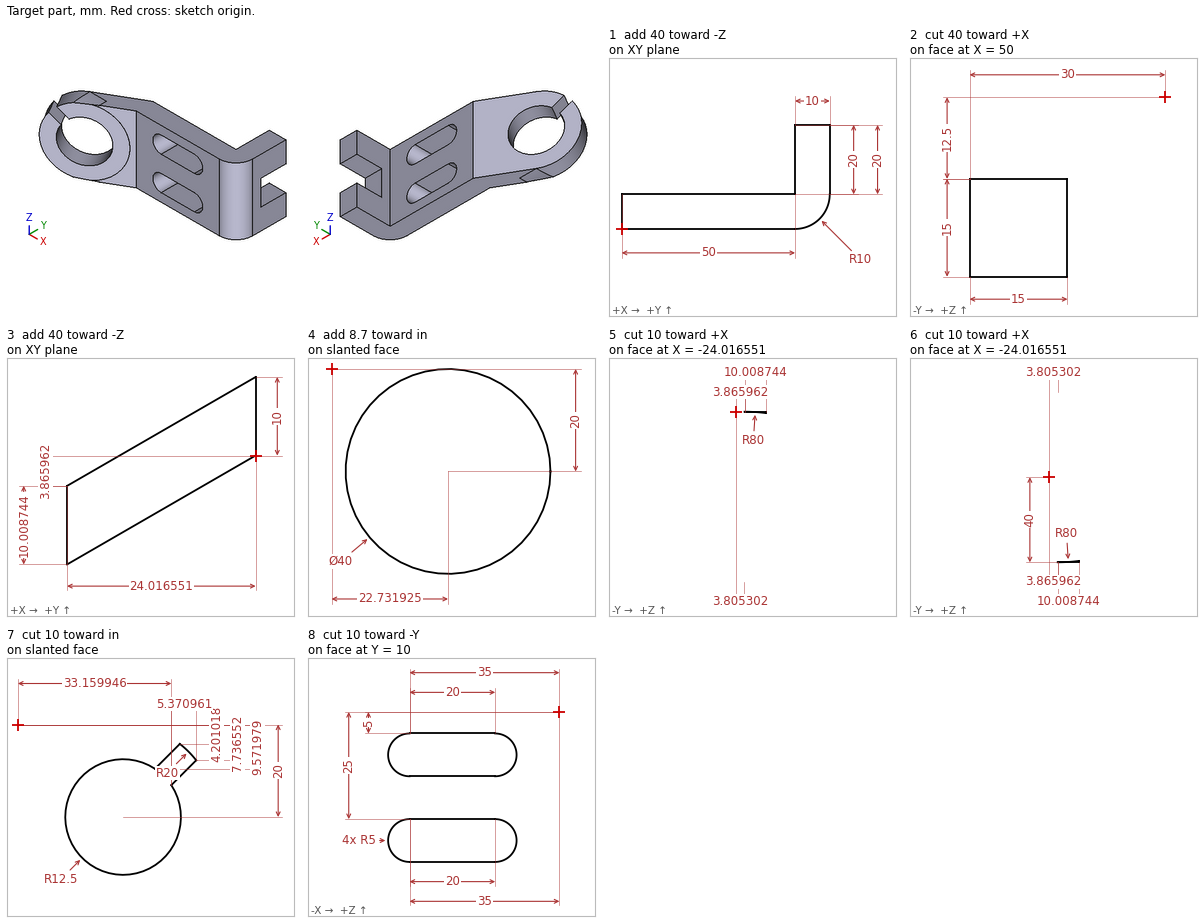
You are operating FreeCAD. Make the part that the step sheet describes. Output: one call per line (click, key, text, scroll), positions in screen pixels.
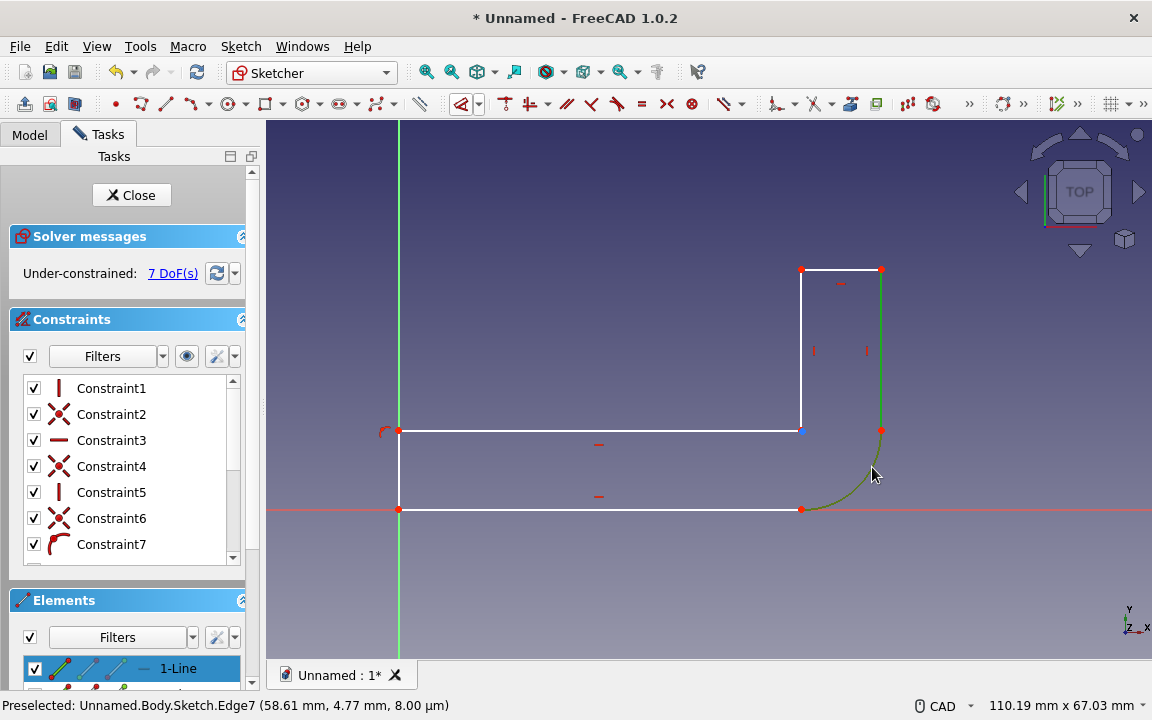
click(617, 104)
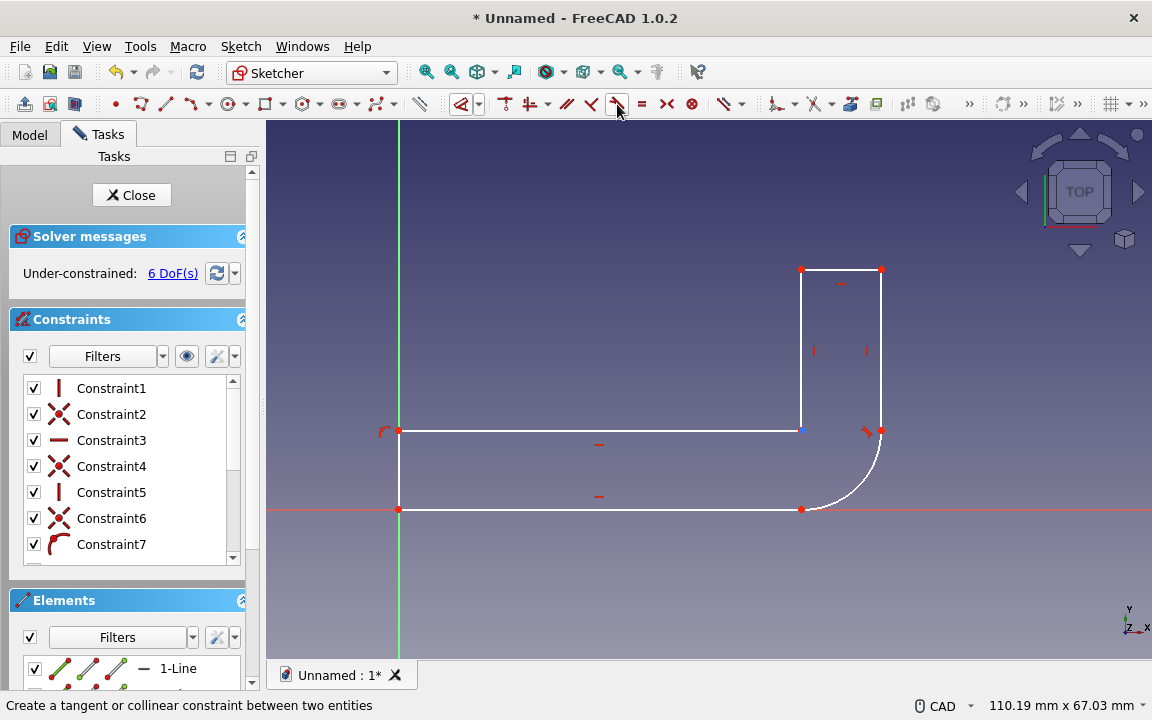
click(519, 510)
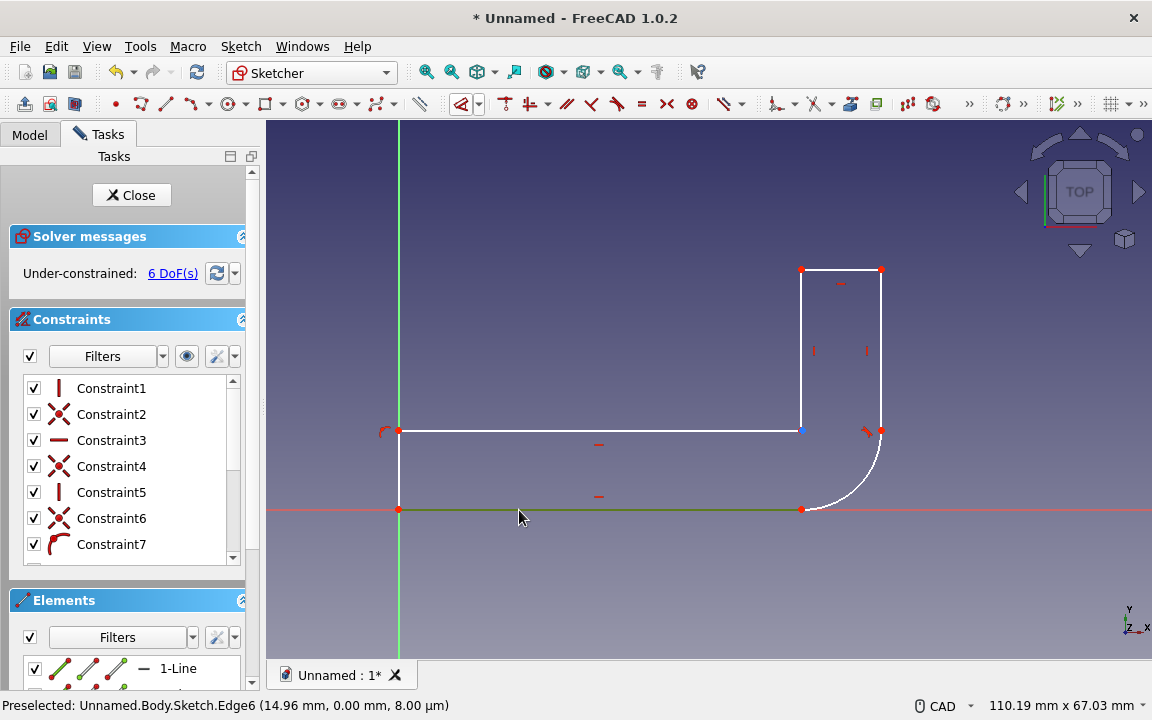
click(872, 467)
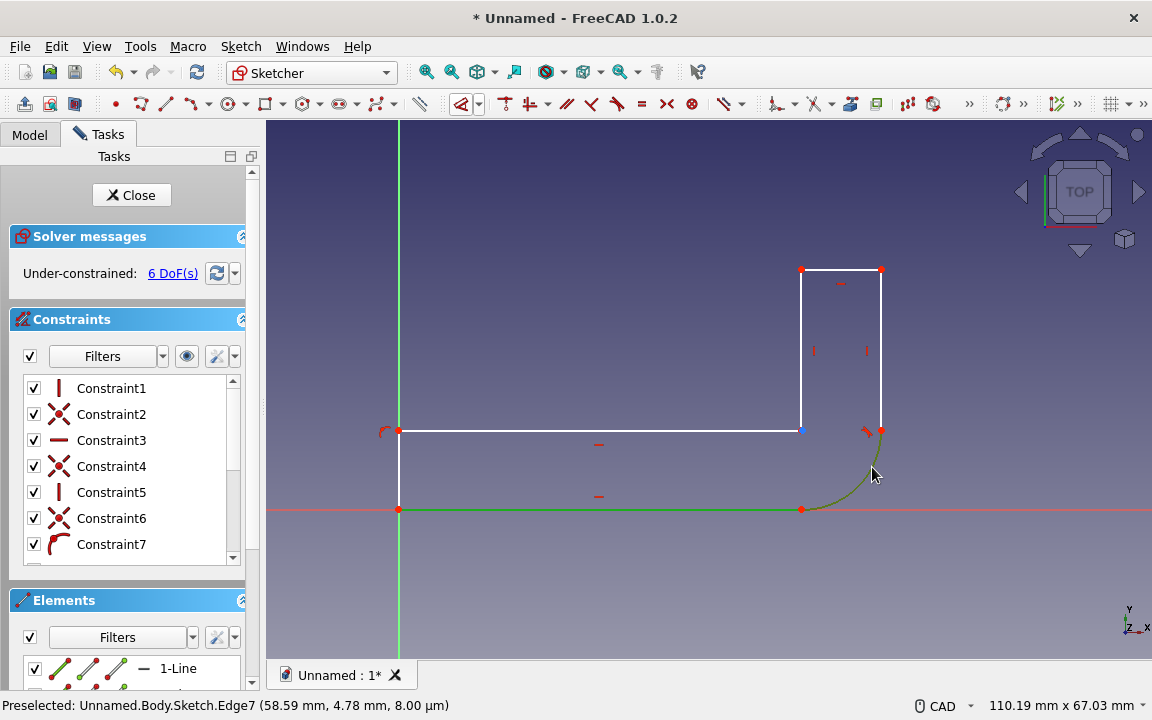
click(617, 104)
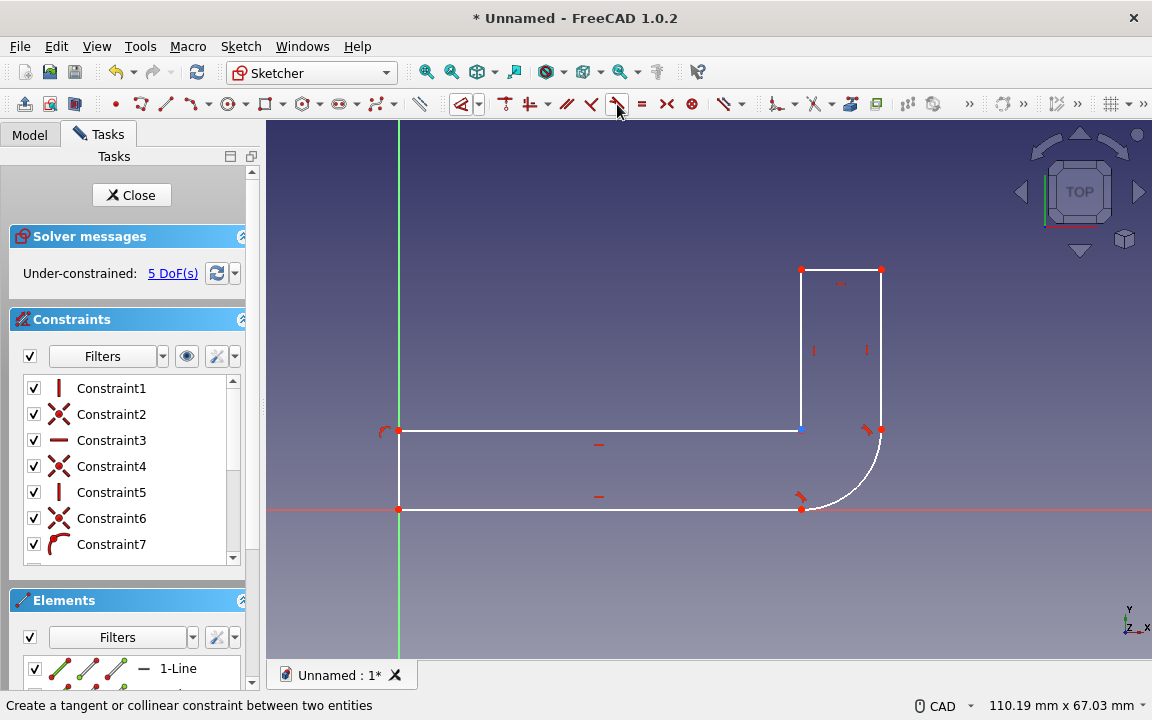
click(872, 466)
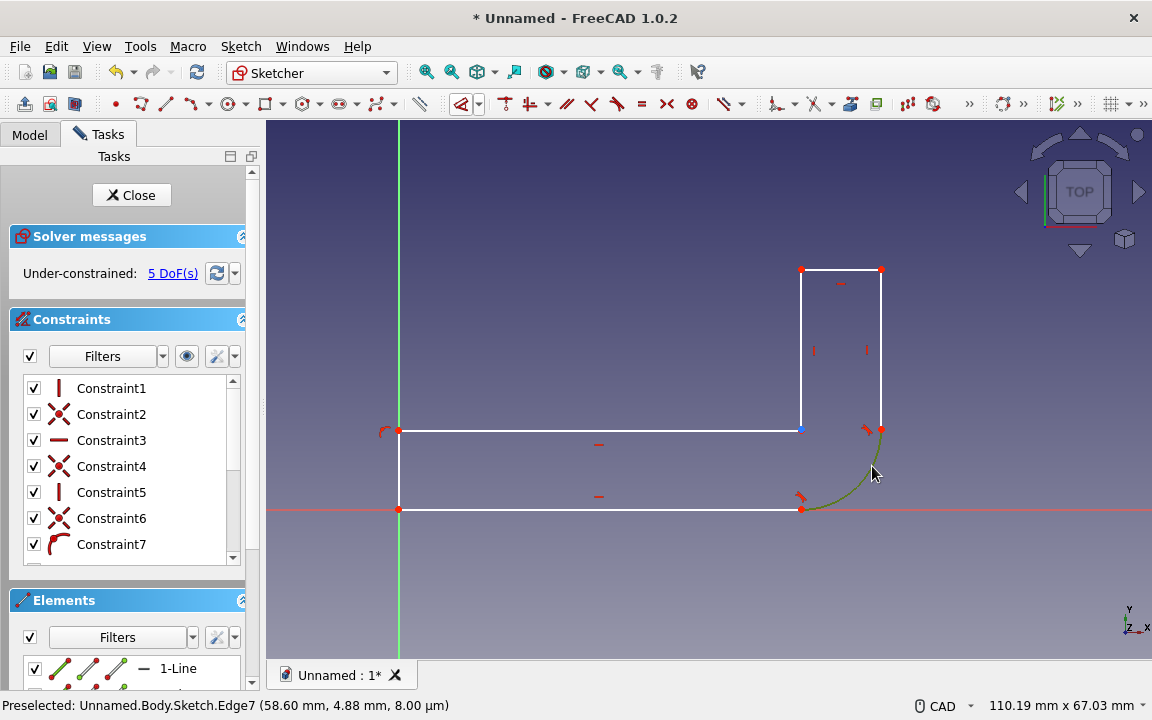
key(k)
key(r)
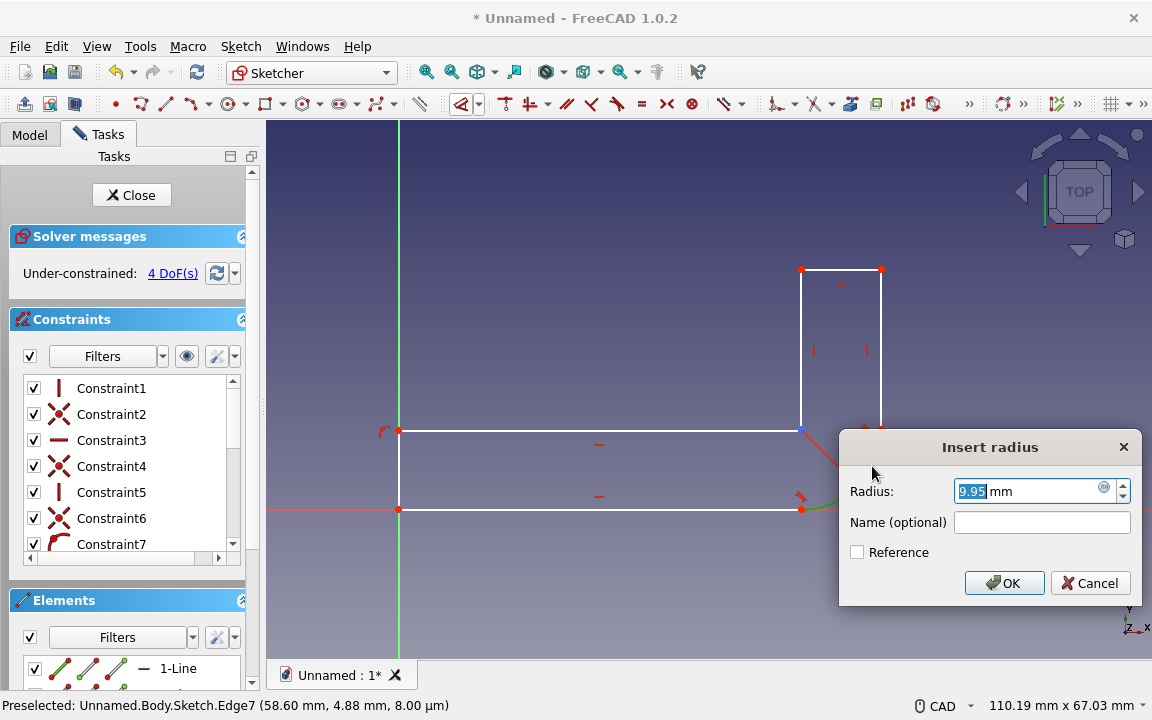
text(10)
key(Return)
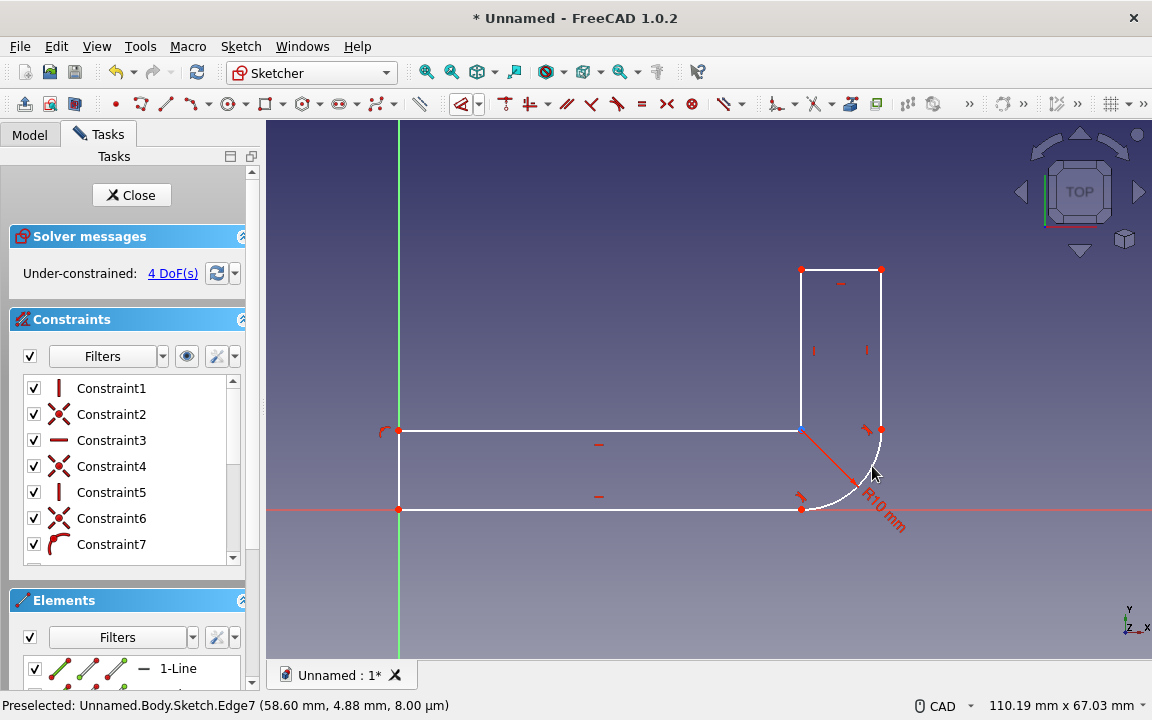
click(881, 382)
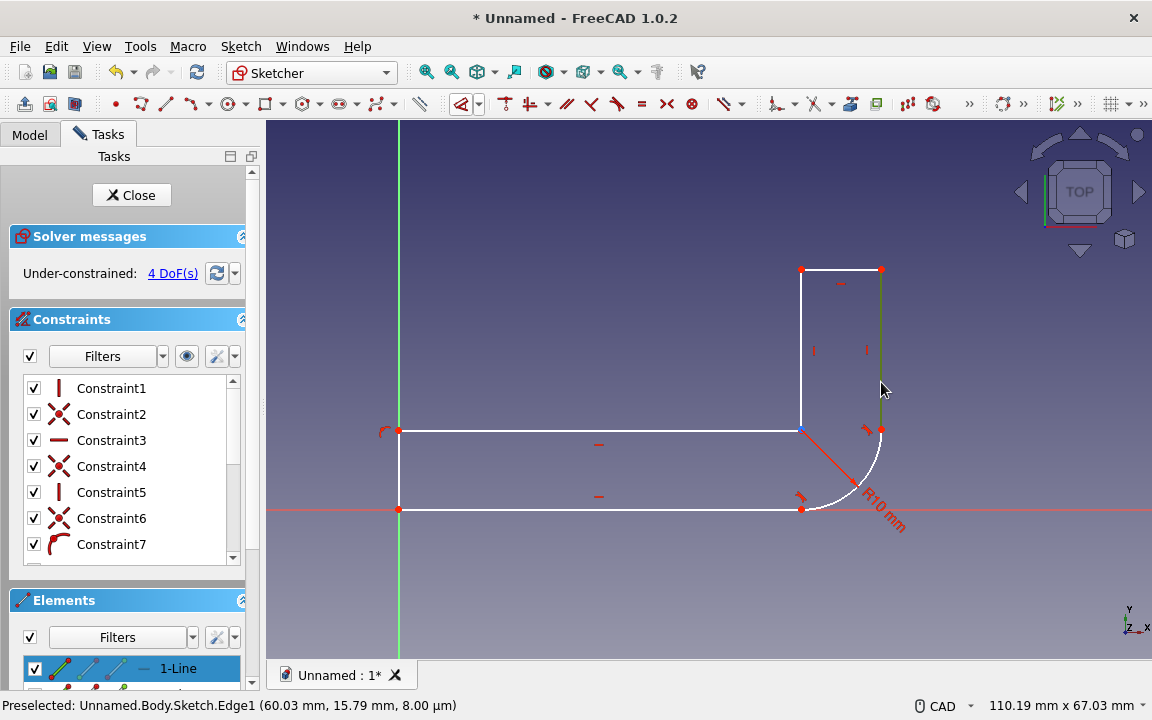
key(i)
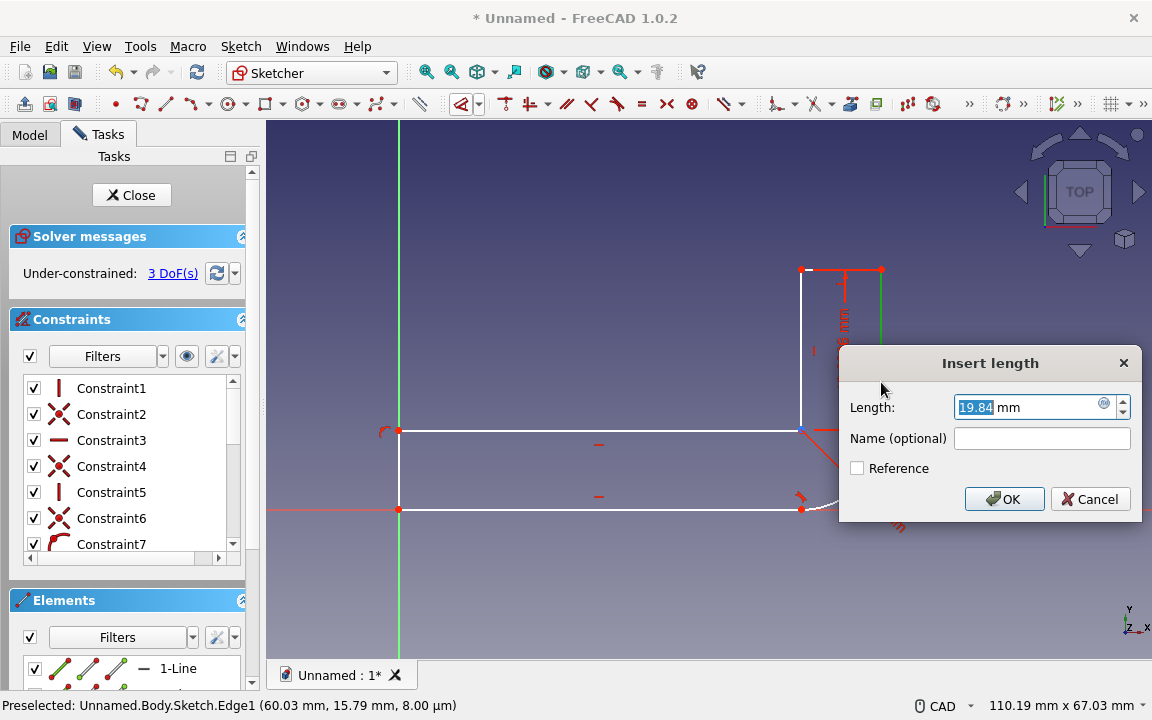
text(20)
key(Return)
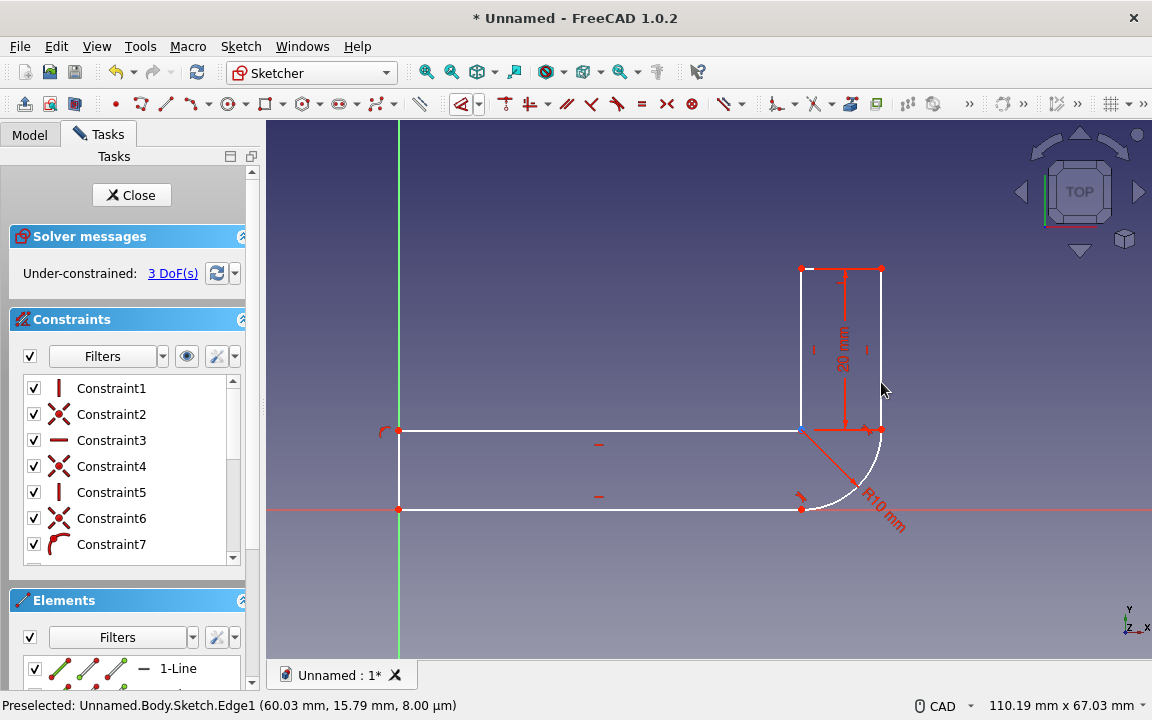
click(857, 269)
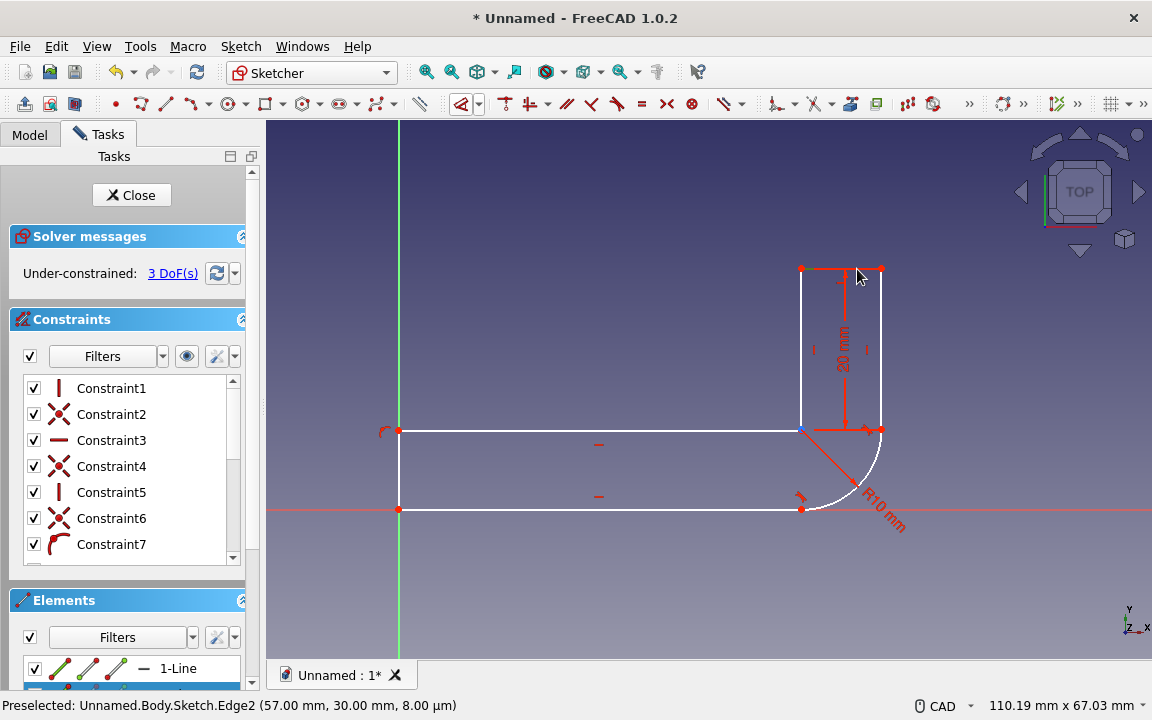
click(478, 104)